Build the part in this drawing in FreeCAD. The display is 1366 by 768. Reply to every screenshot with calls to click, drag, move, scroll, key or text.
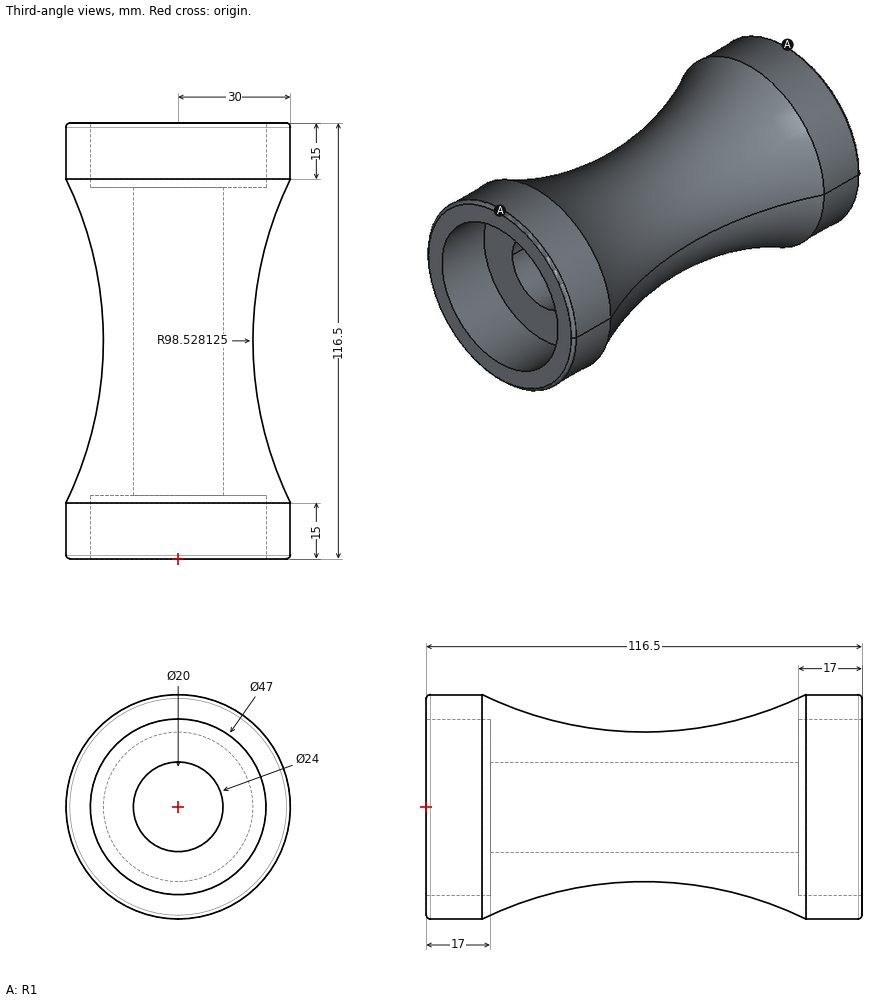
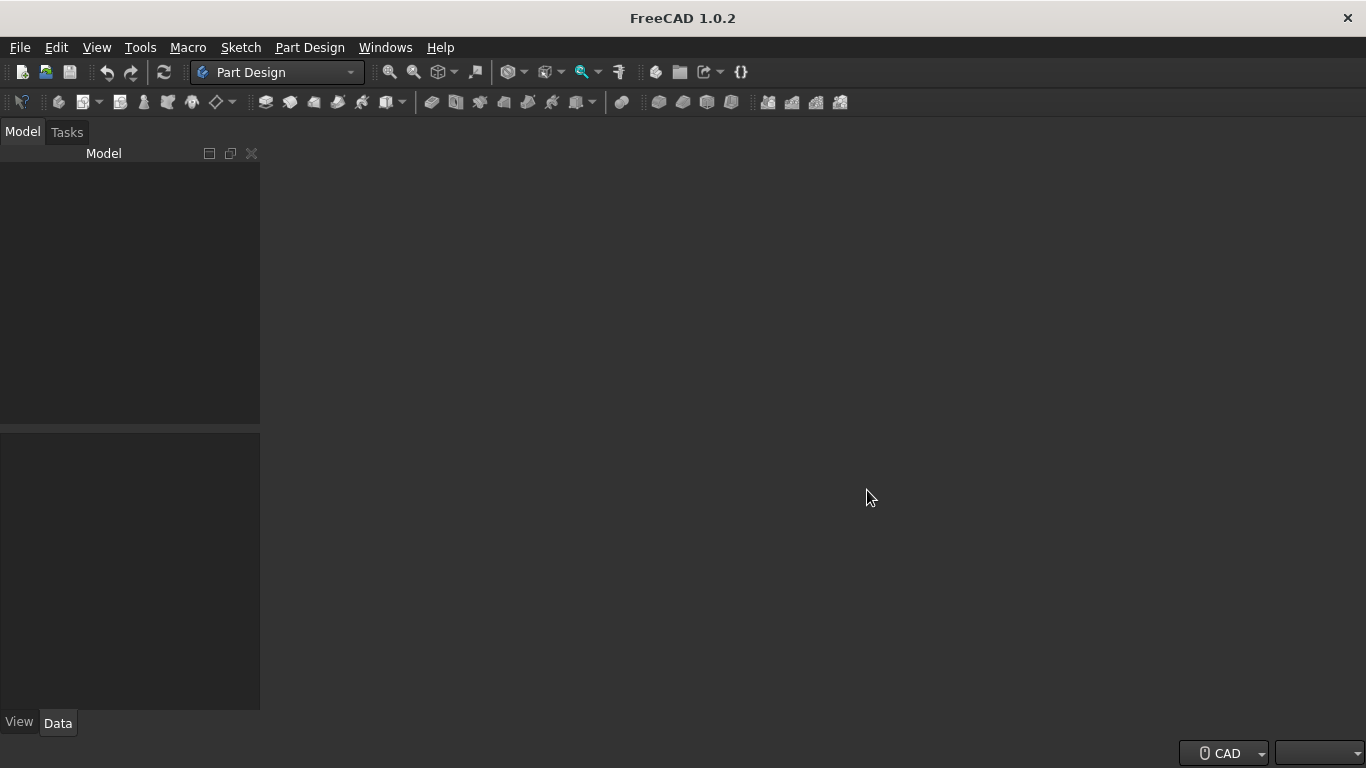
click(22, 72)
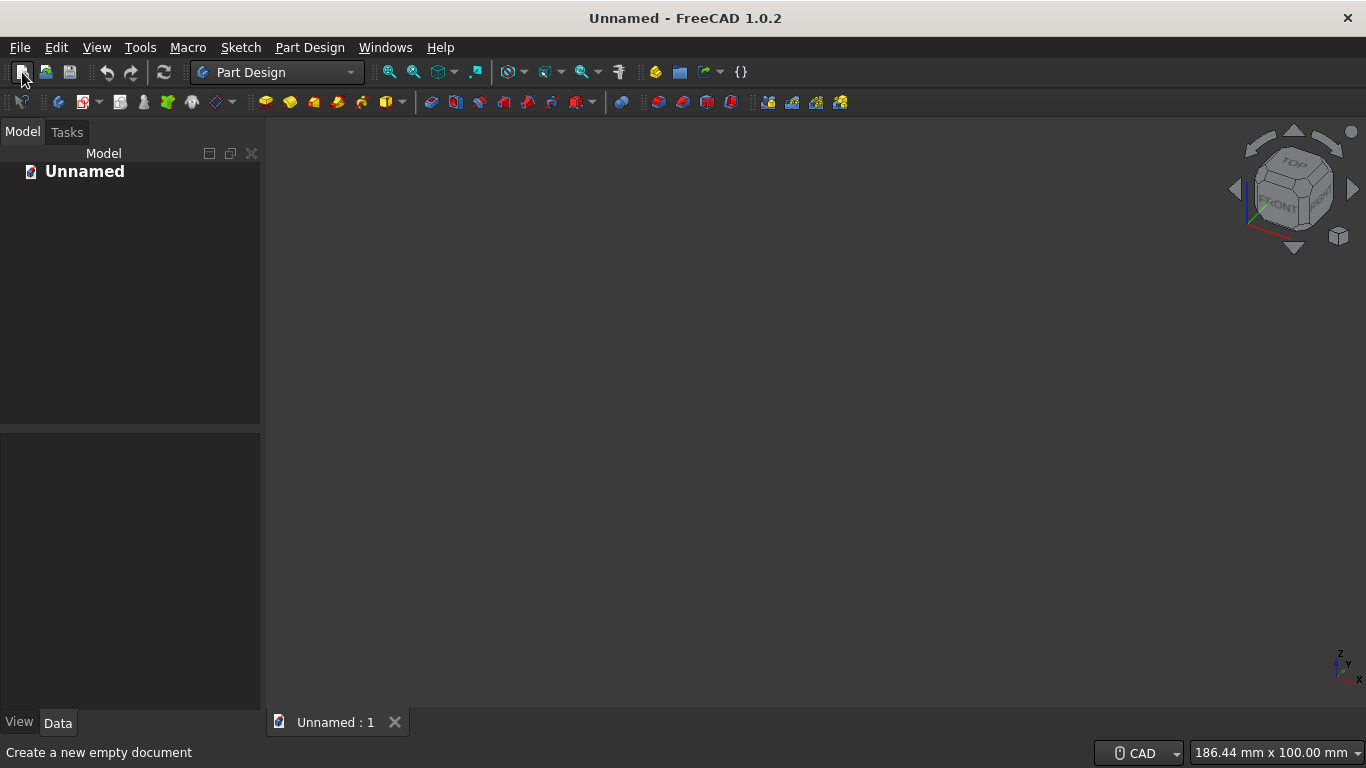
click(84, 102)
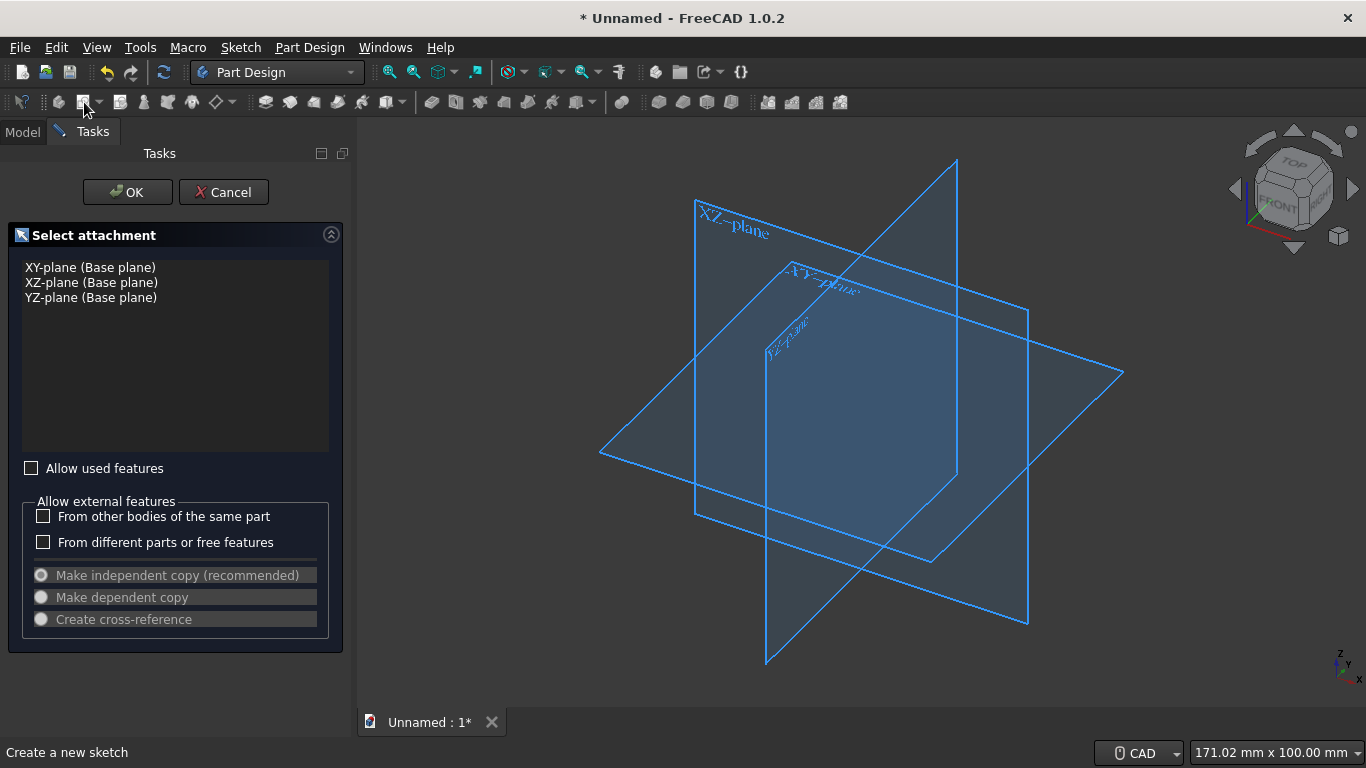
click(82, 268)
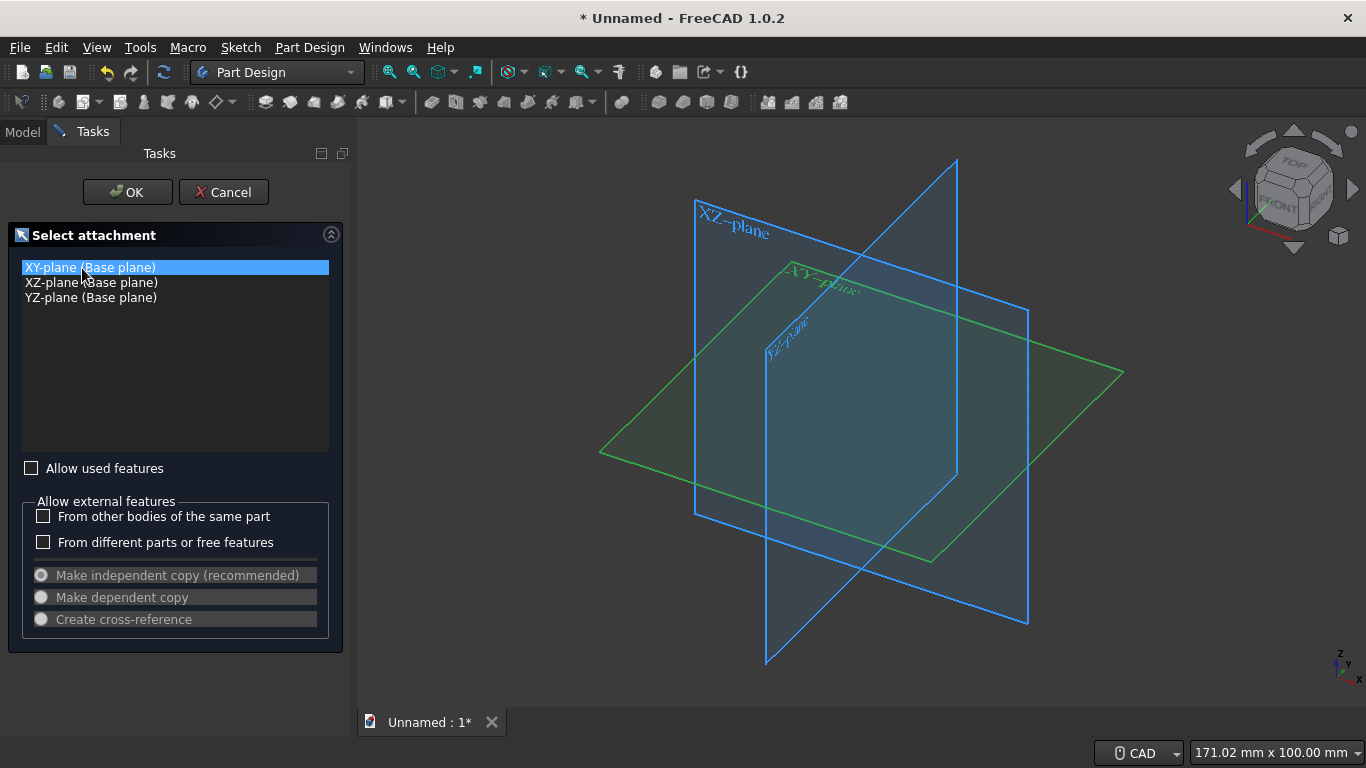
click(128, 192)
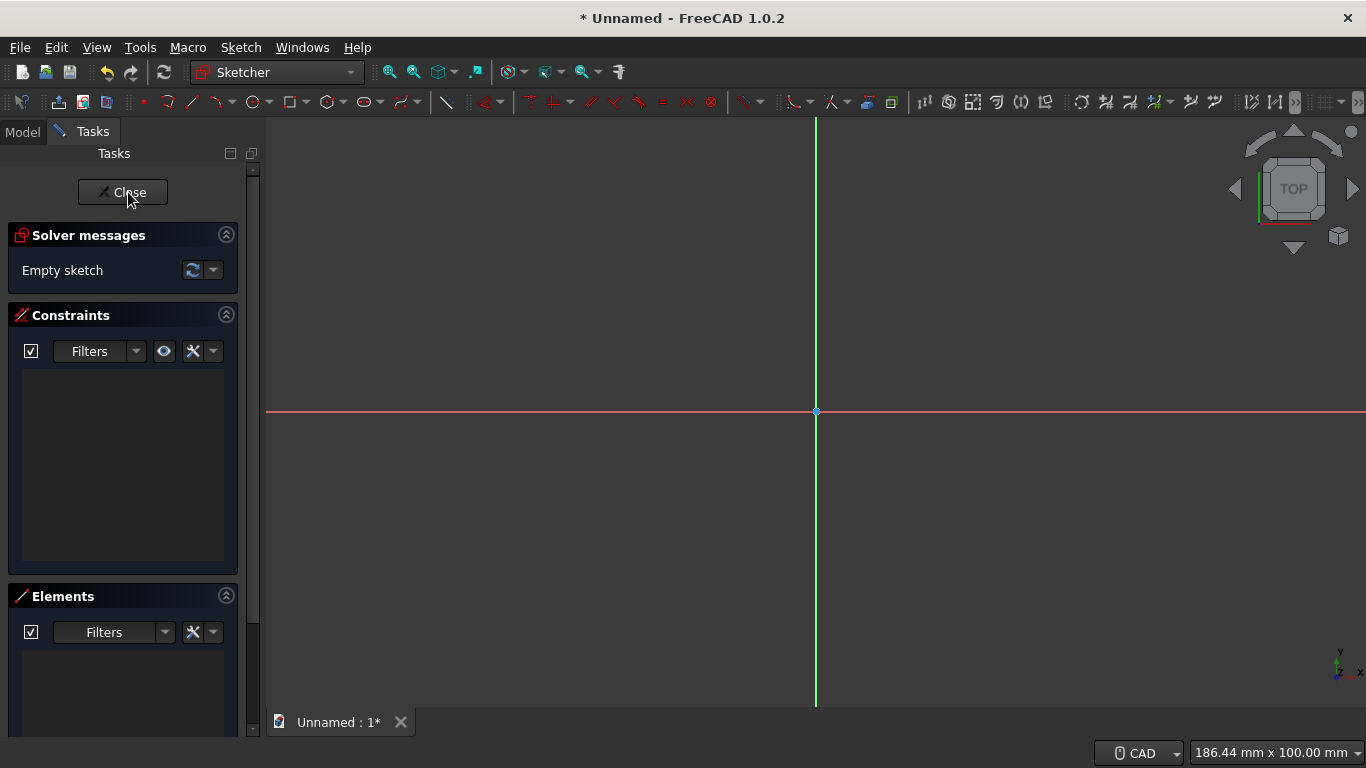
scroll(619, 679, down, 4)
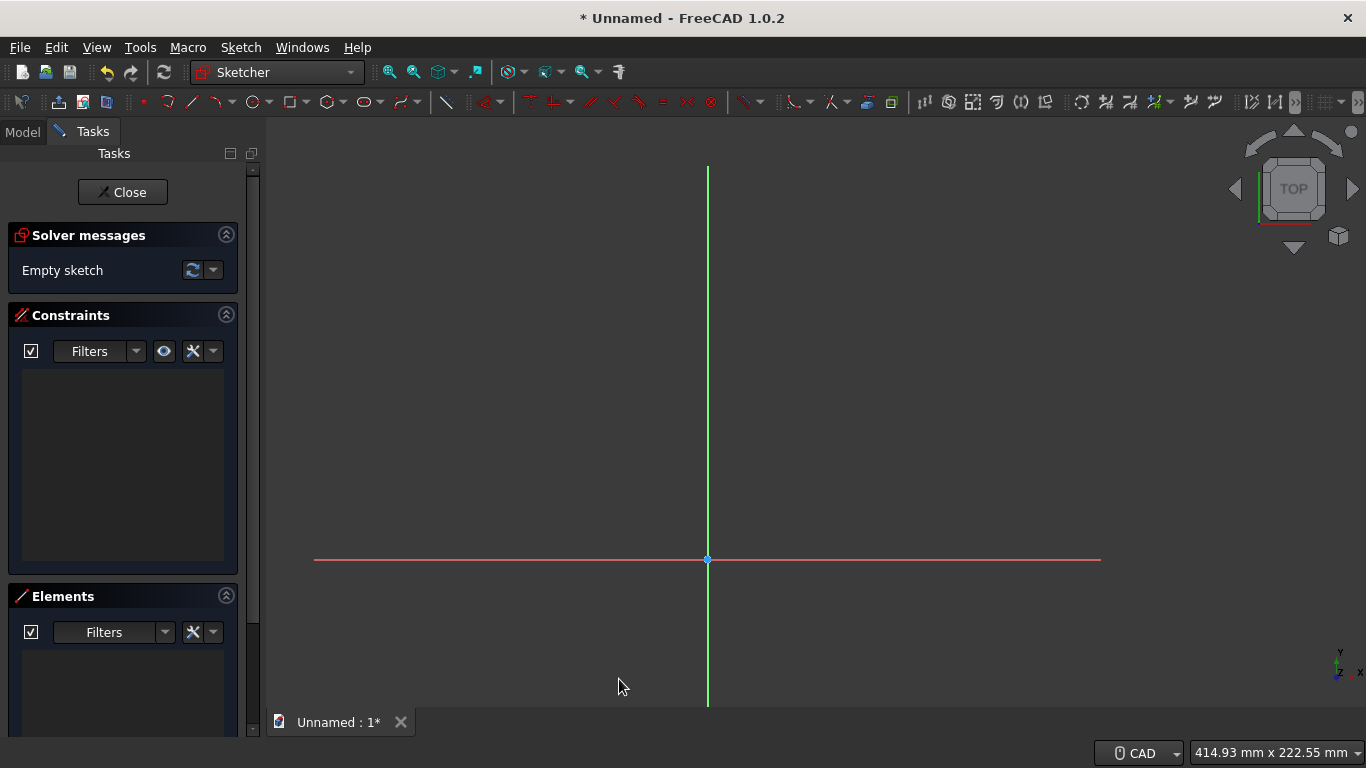
click(168, 102)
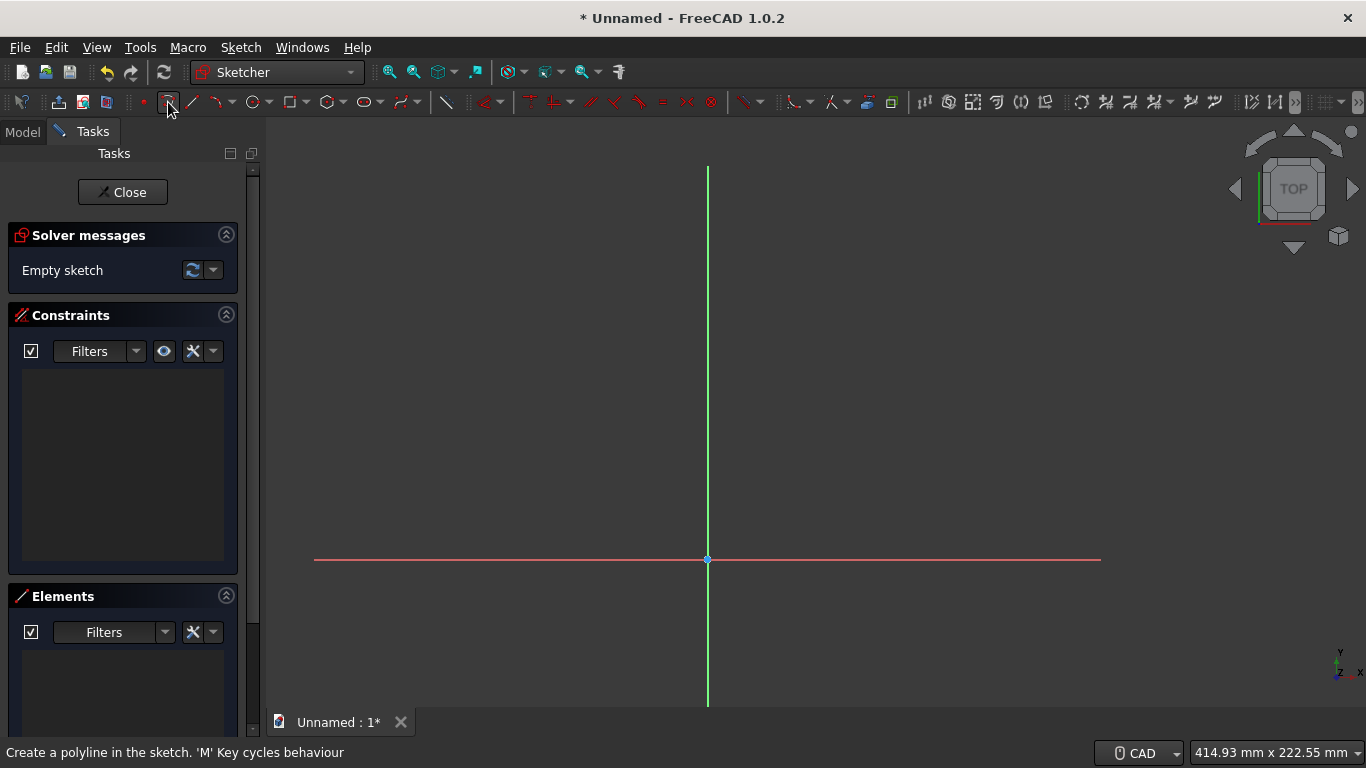
click(787, 290)
click(787, 251)
click(708, 251)
click(708, 560)
click(787, 551)
click(787, 520)
right_click(787, 520)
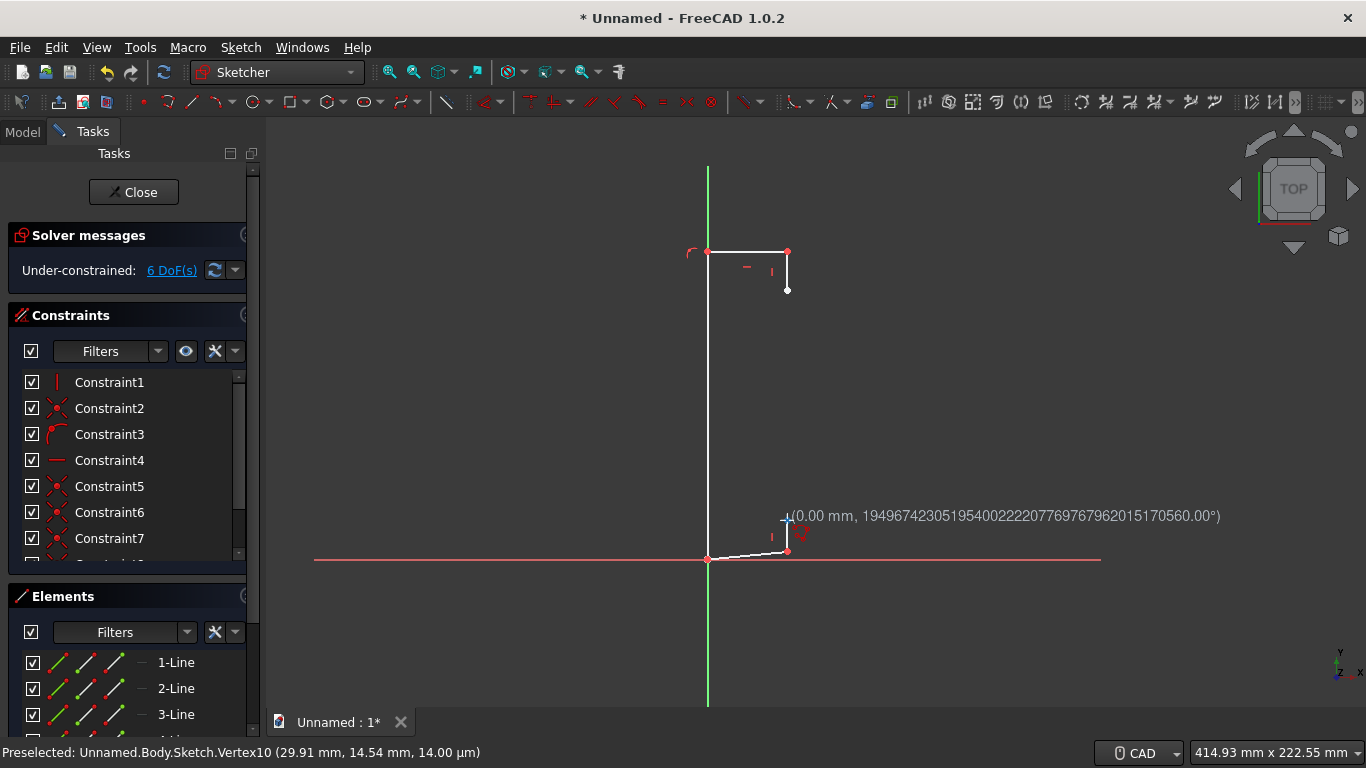
click(216, 102)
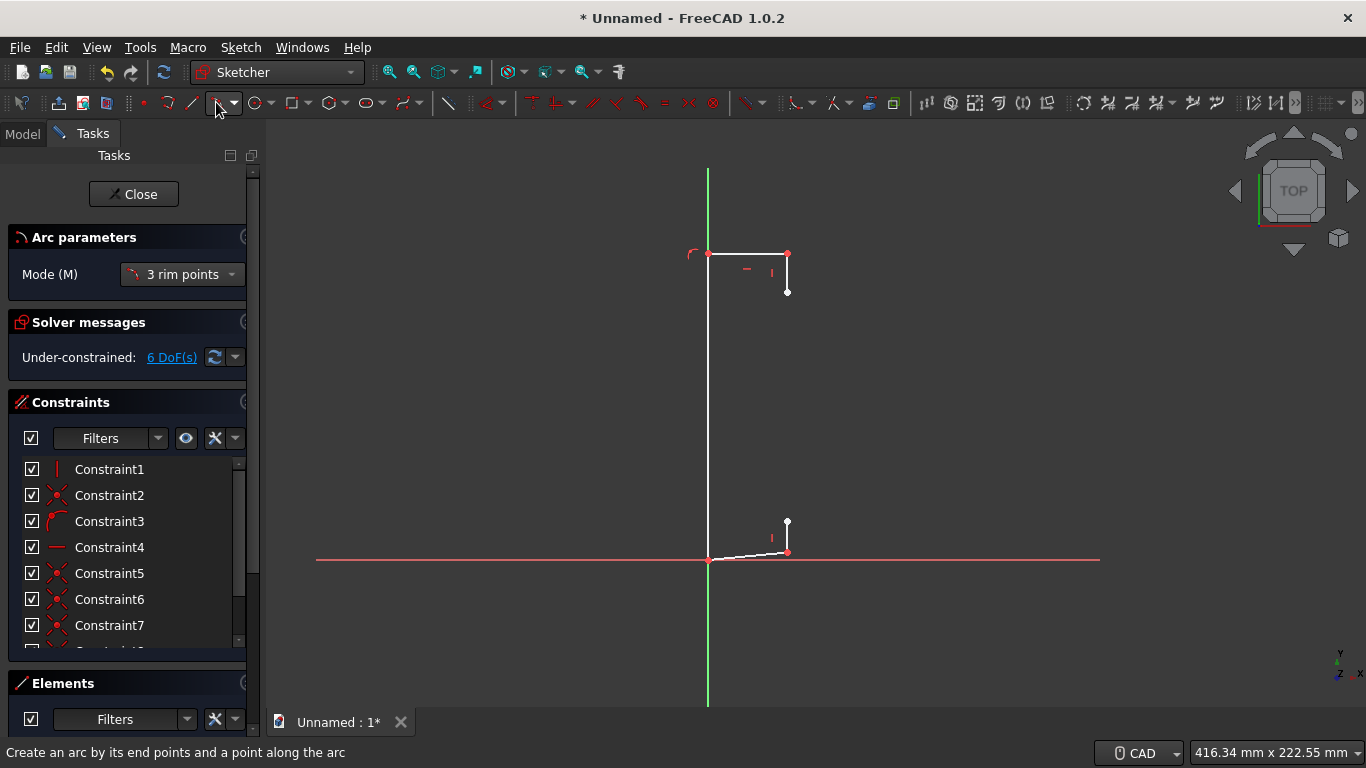
click(787, 522)
click(787, 292)
click(761, 406)
key(Escape)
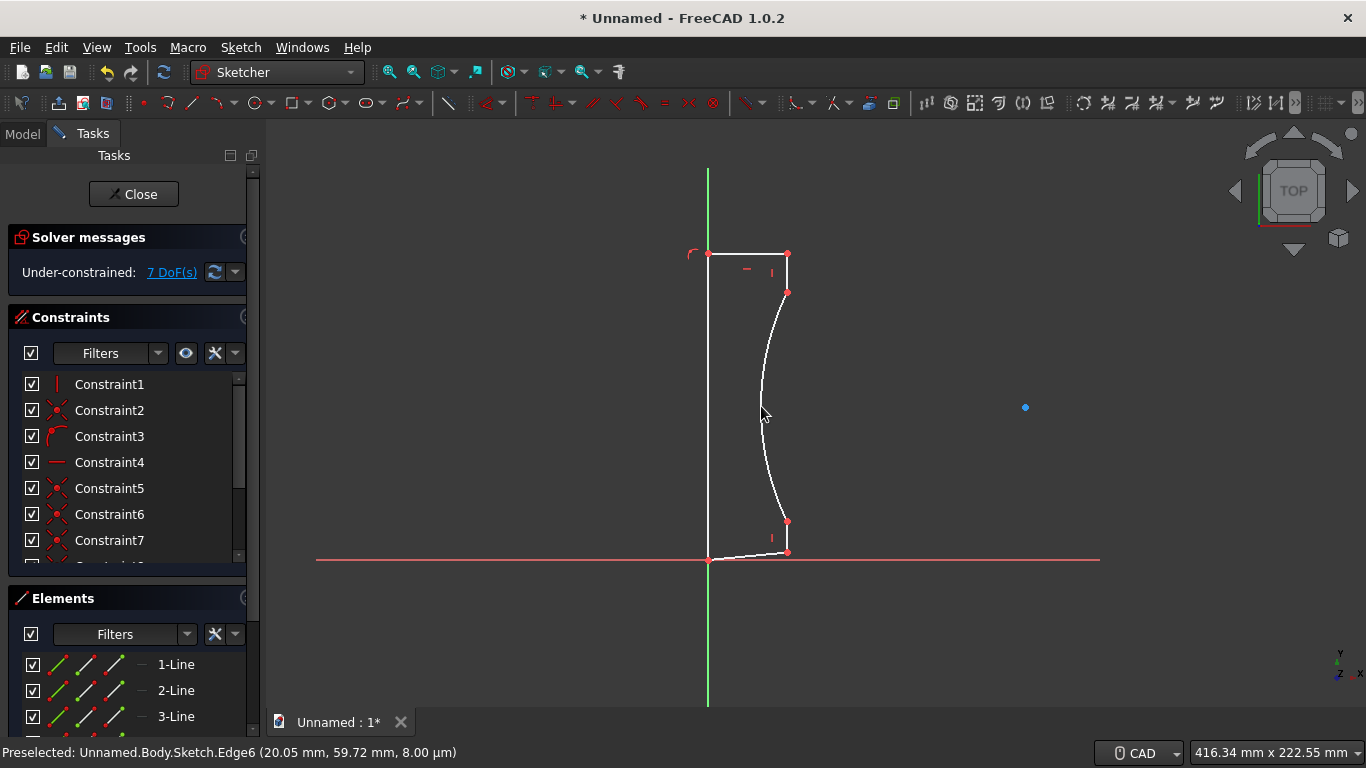
click(732, 558)